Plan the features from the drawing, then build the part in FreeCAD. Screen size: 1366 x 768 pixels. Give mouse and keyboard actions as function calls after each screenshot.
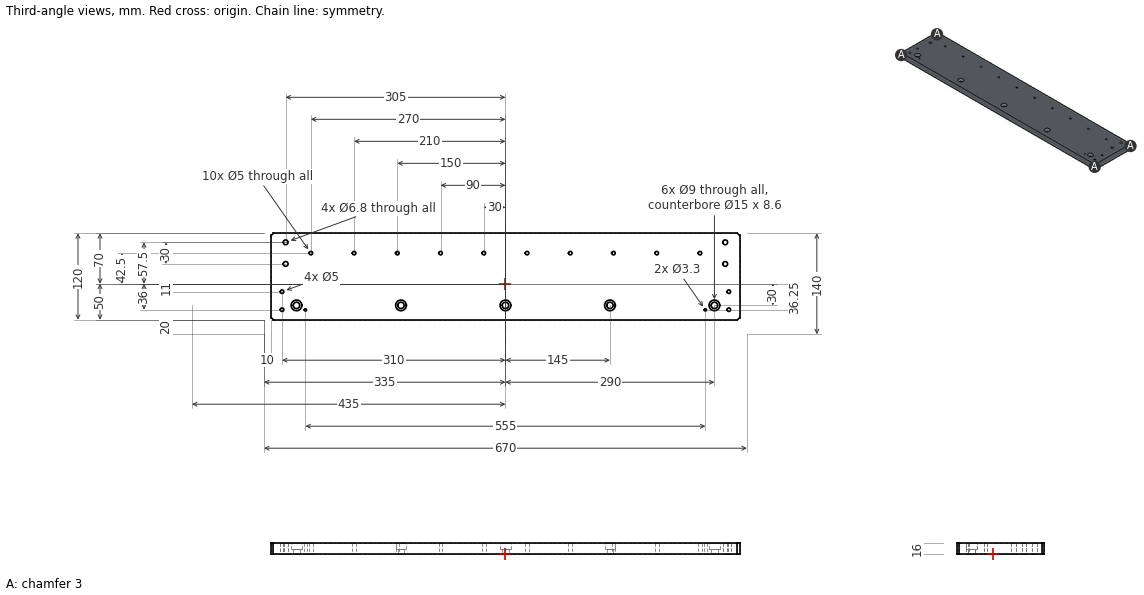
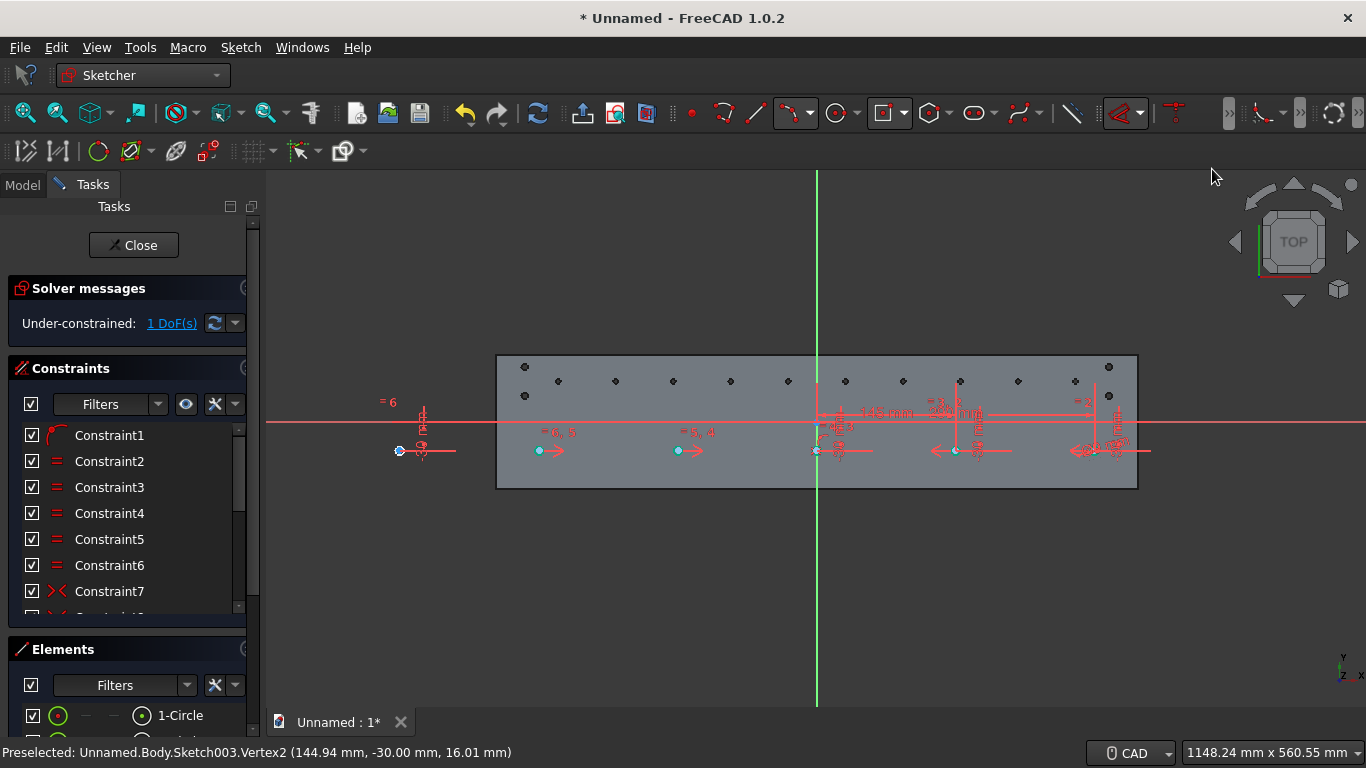
click(400, 451)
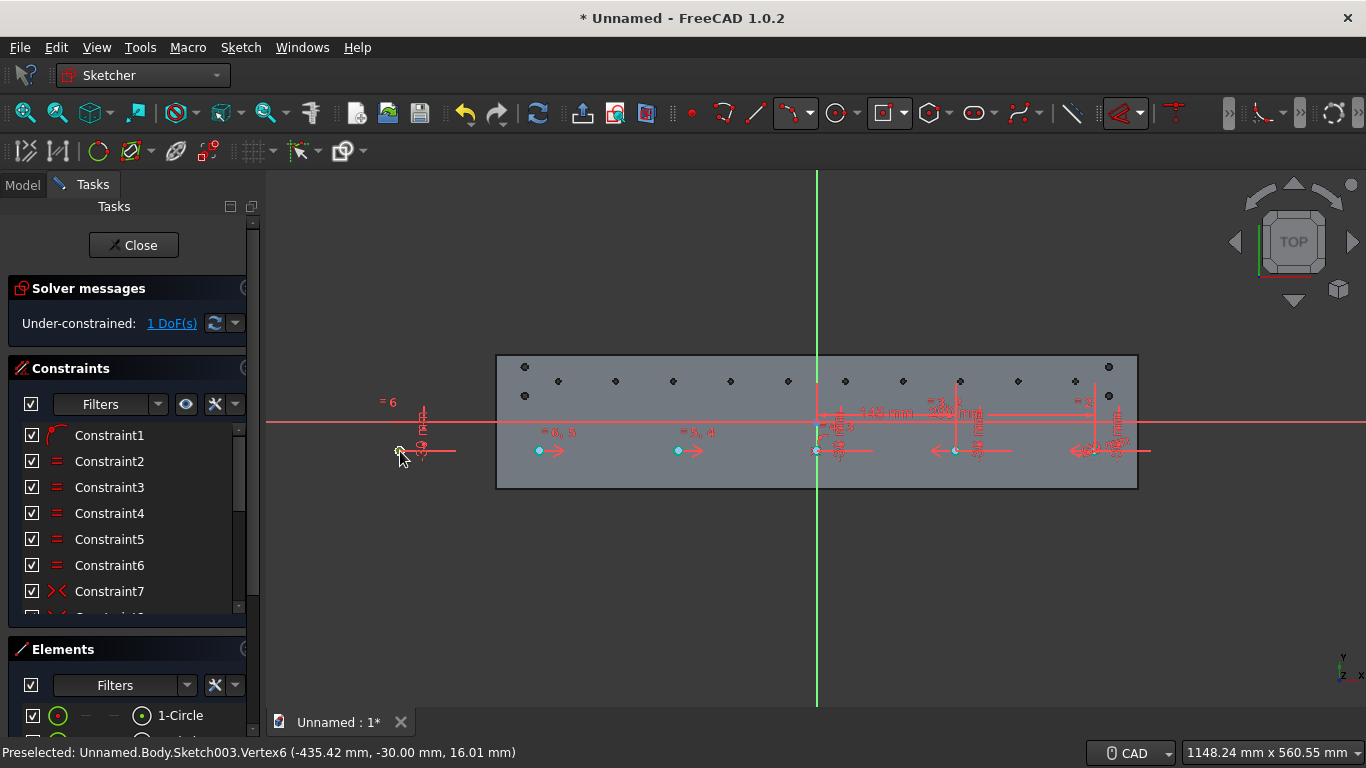
click(1142, 114)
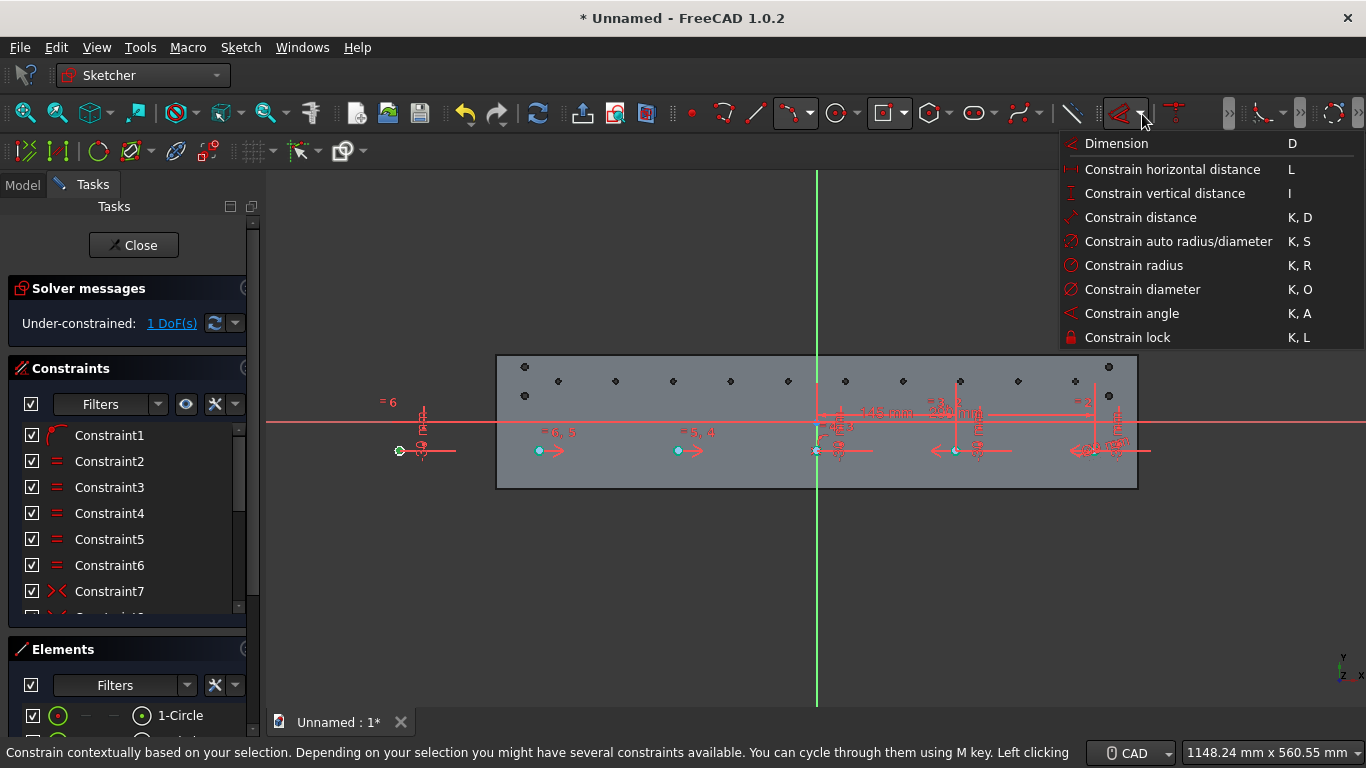
click(1212, 169)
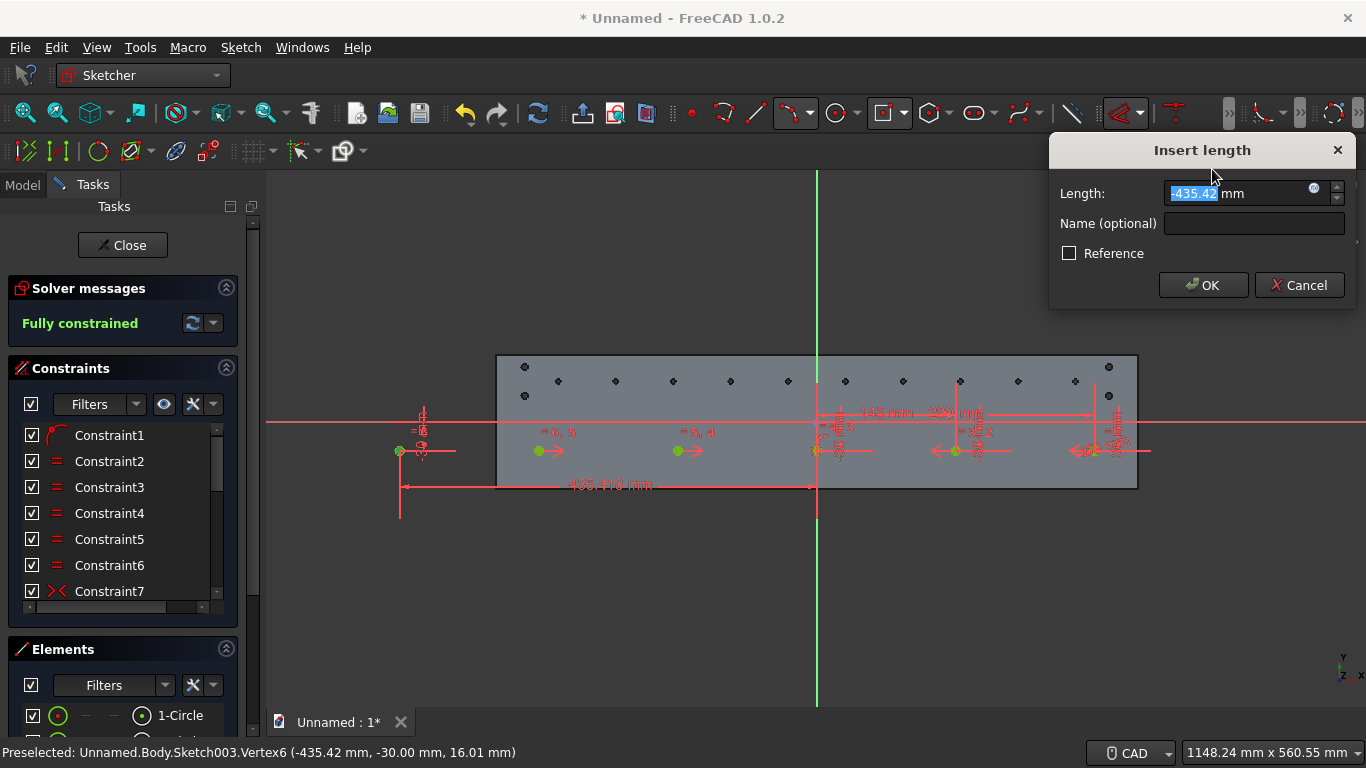
text(-435)
key(Return)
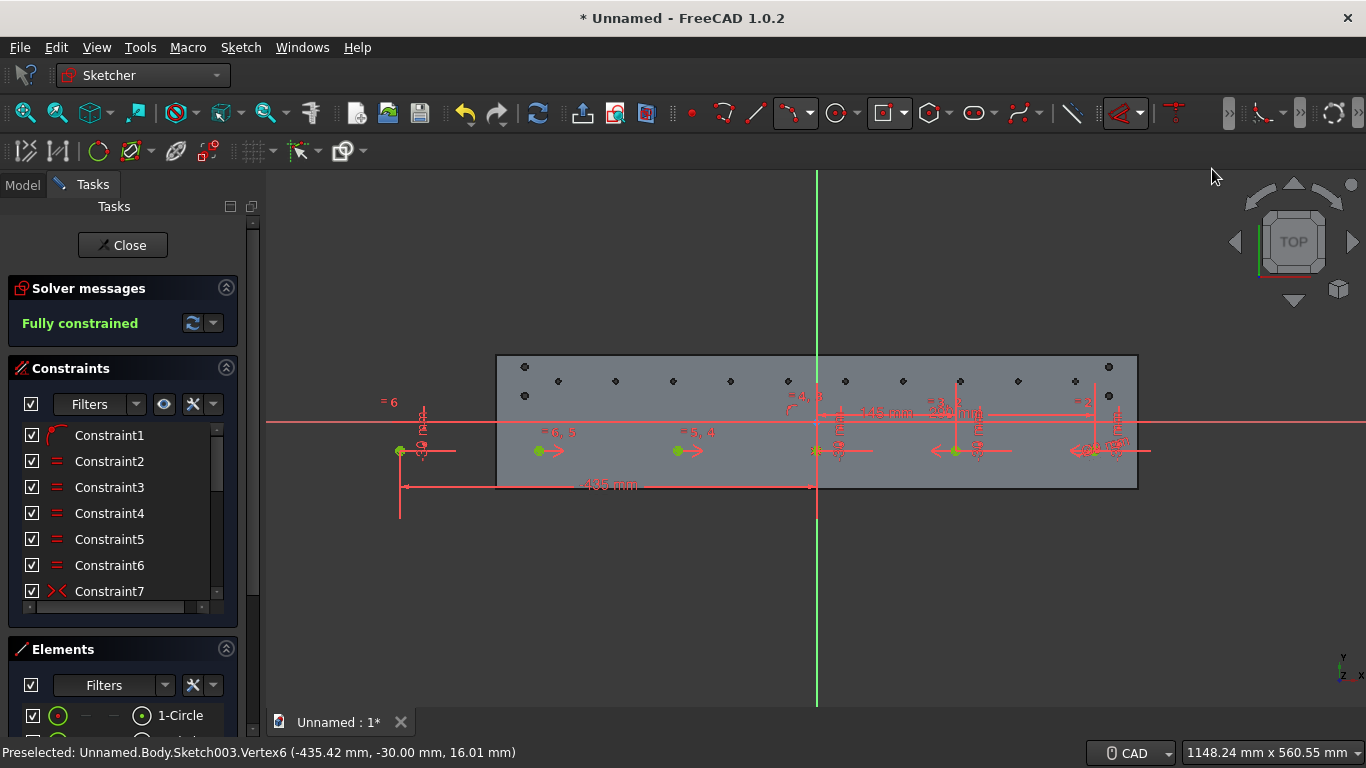
click(123, 245)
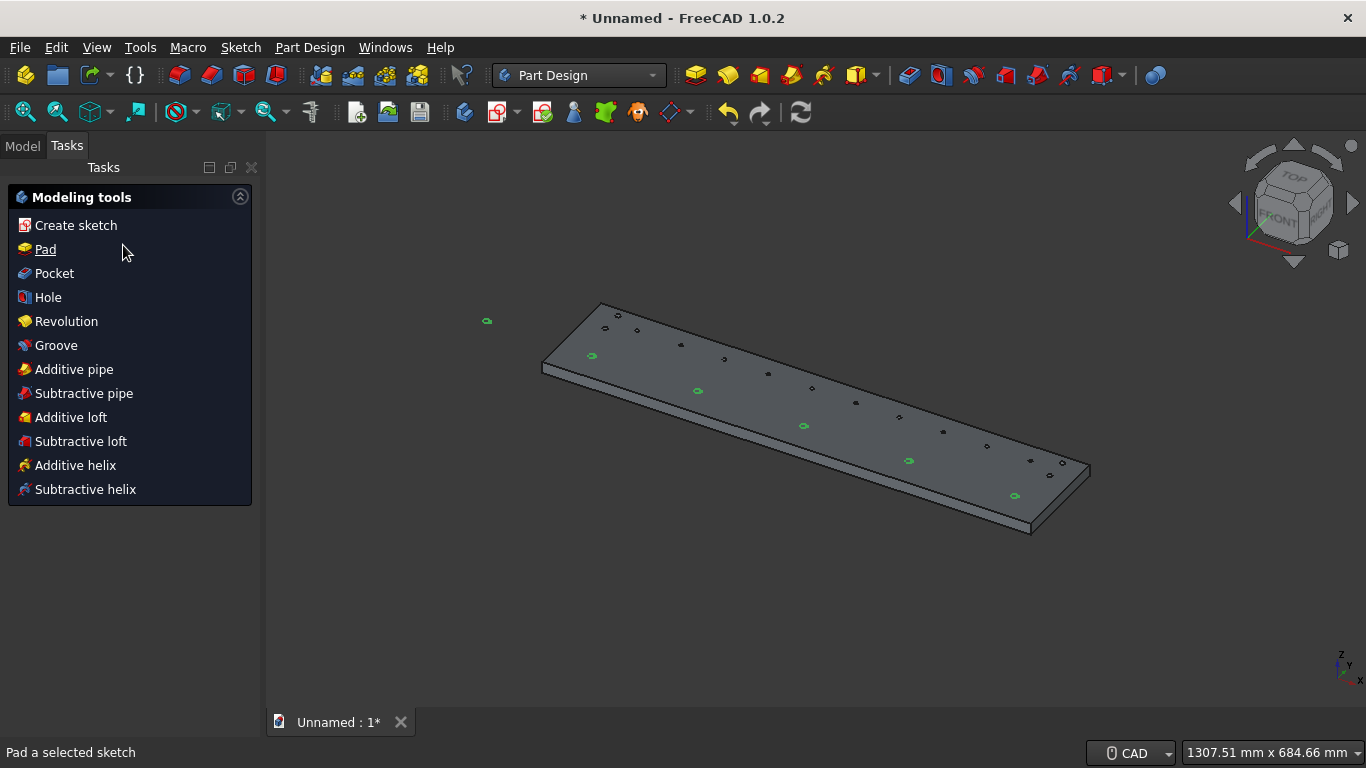
click(942, 76)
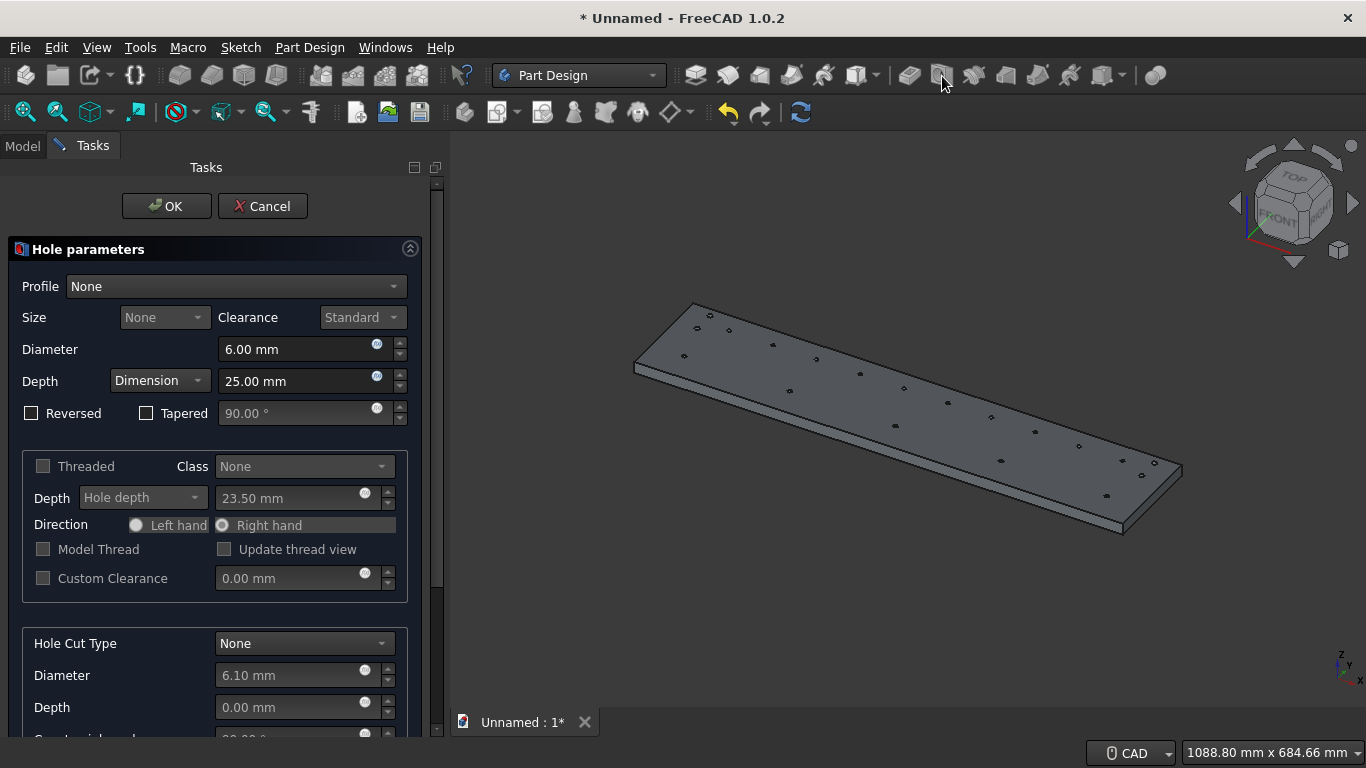
triple_click(305, 349)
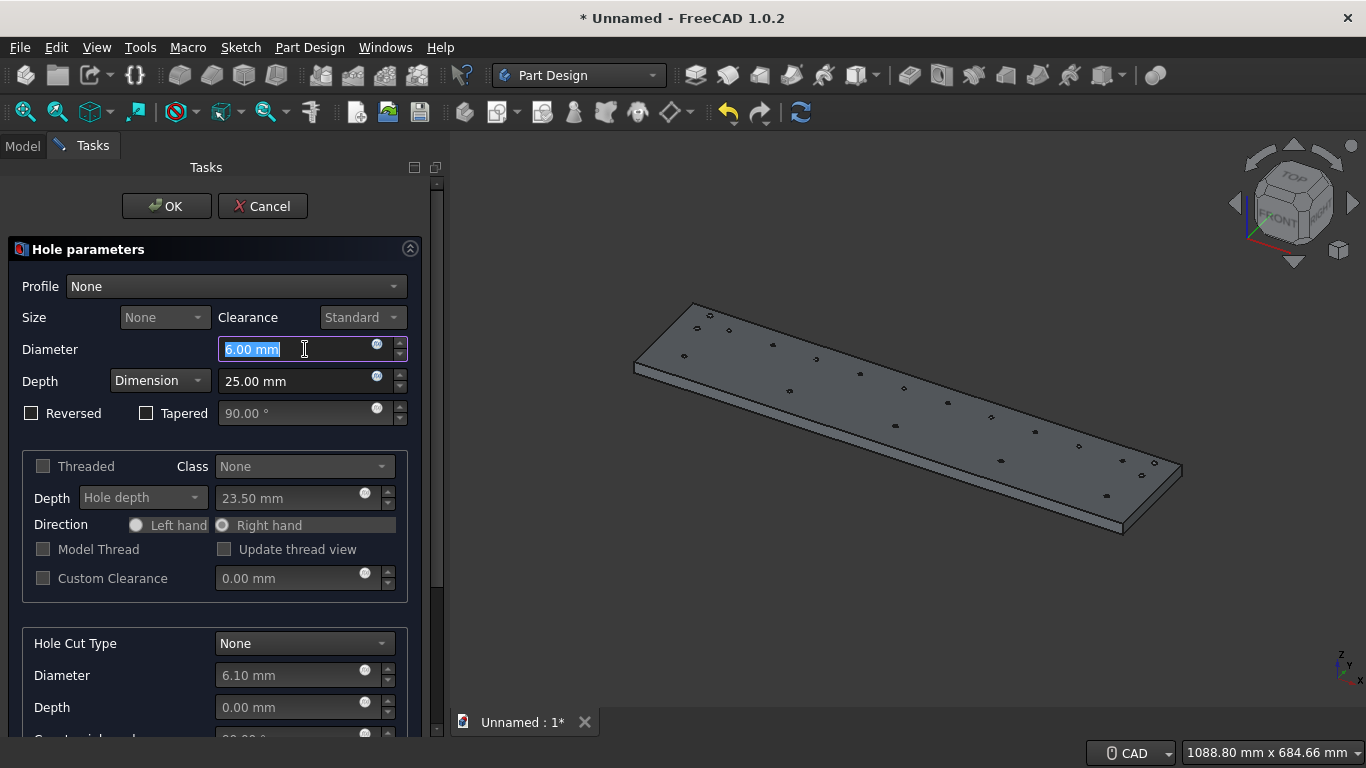
text(9)
key(Tab)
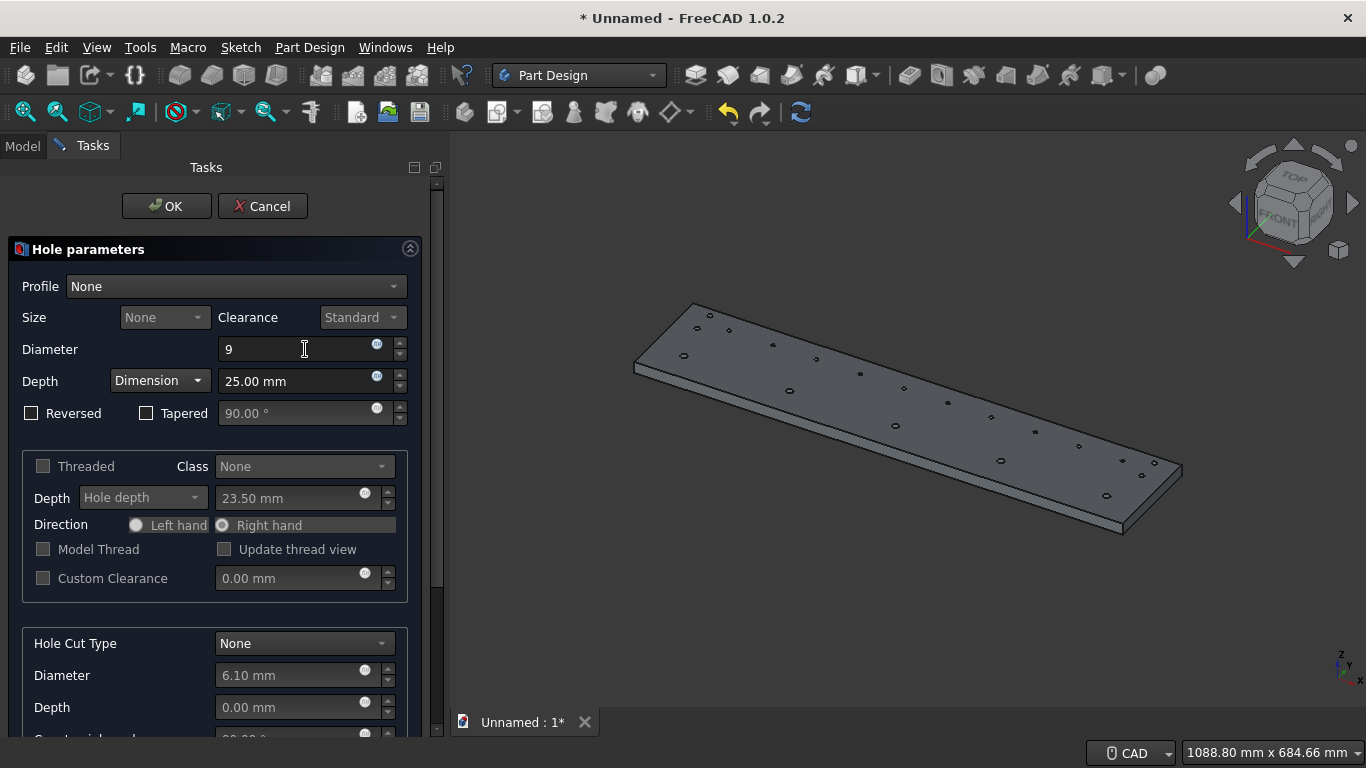
click(161, 380)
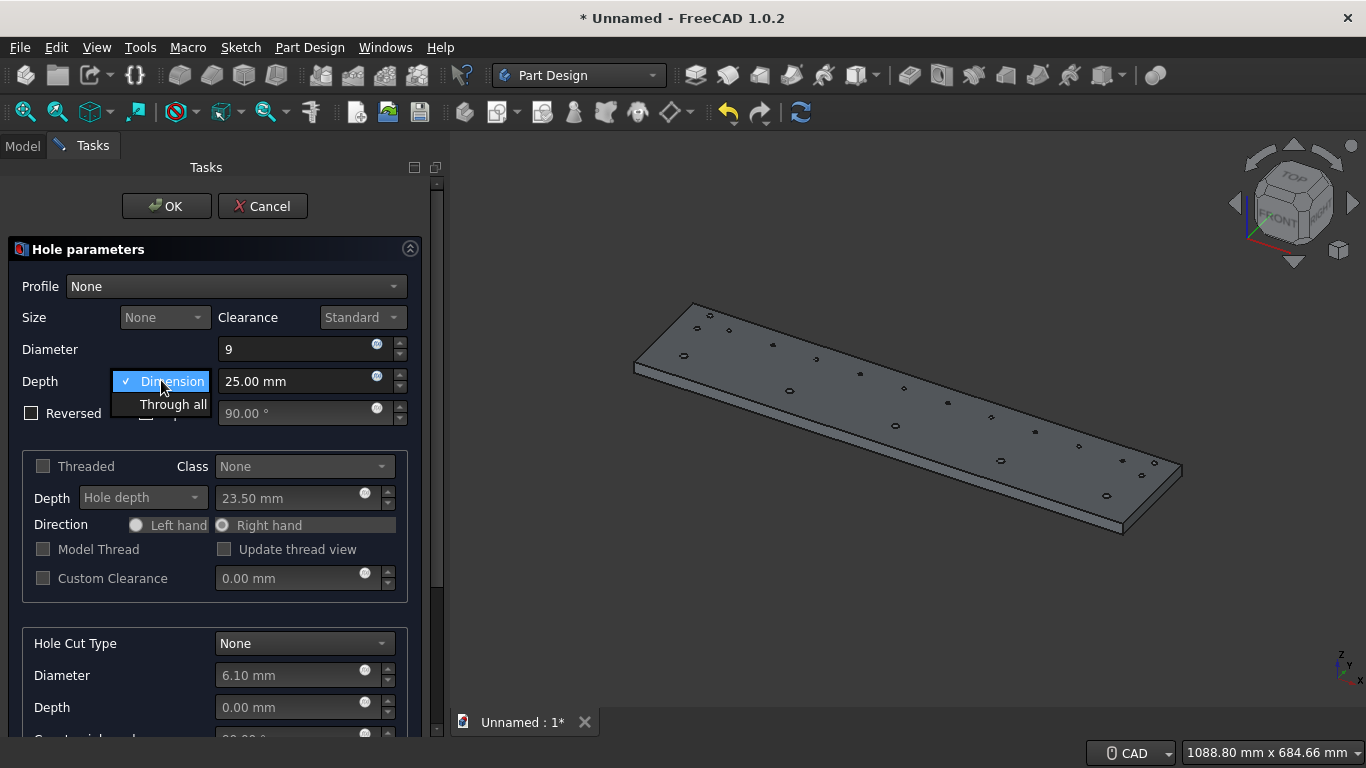
click(160, 404)